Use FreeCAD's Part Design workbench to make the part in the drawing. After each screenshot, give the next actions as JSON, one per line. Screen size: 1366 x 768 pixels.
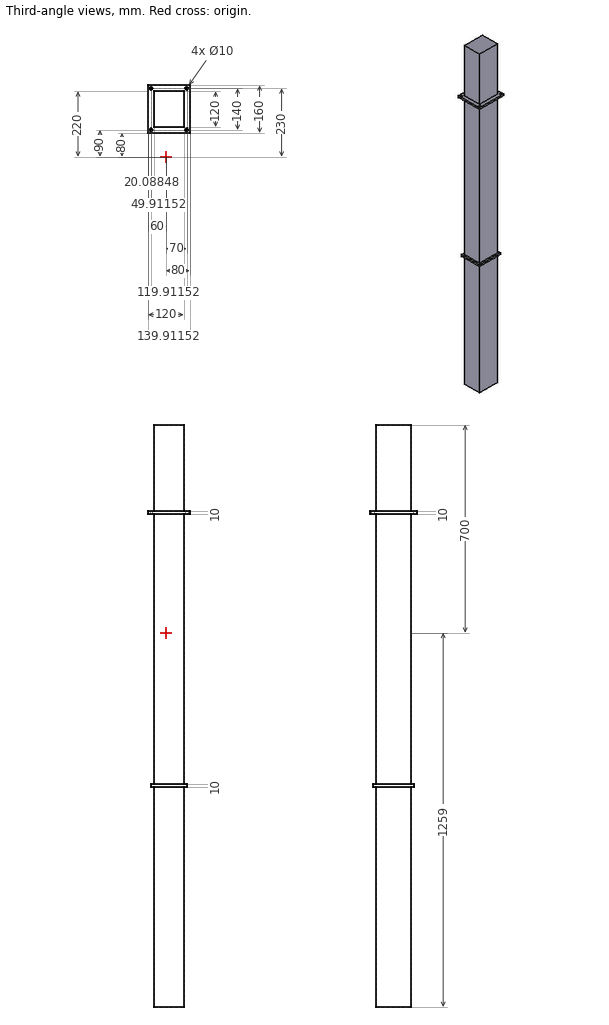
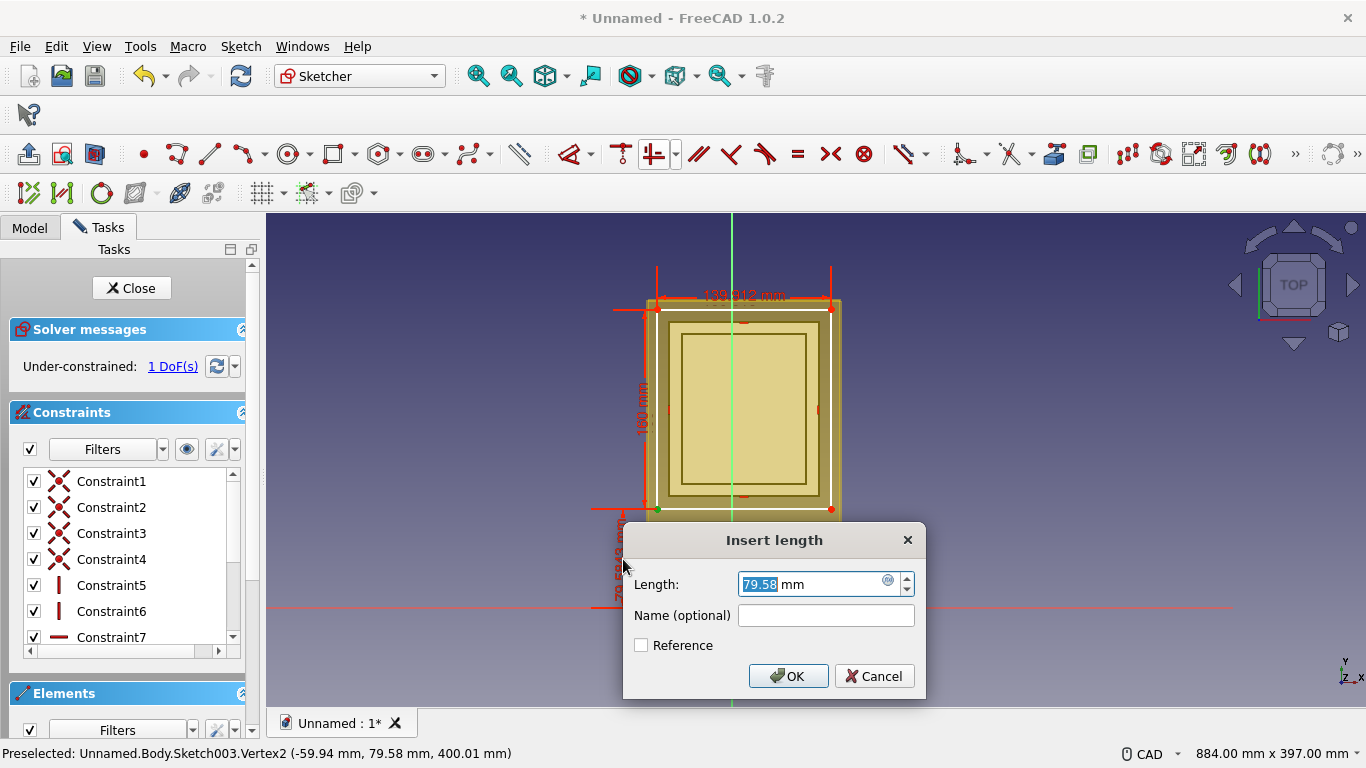
{"action": "type", "text": "80"}
{"action": "key", "text": "Return"}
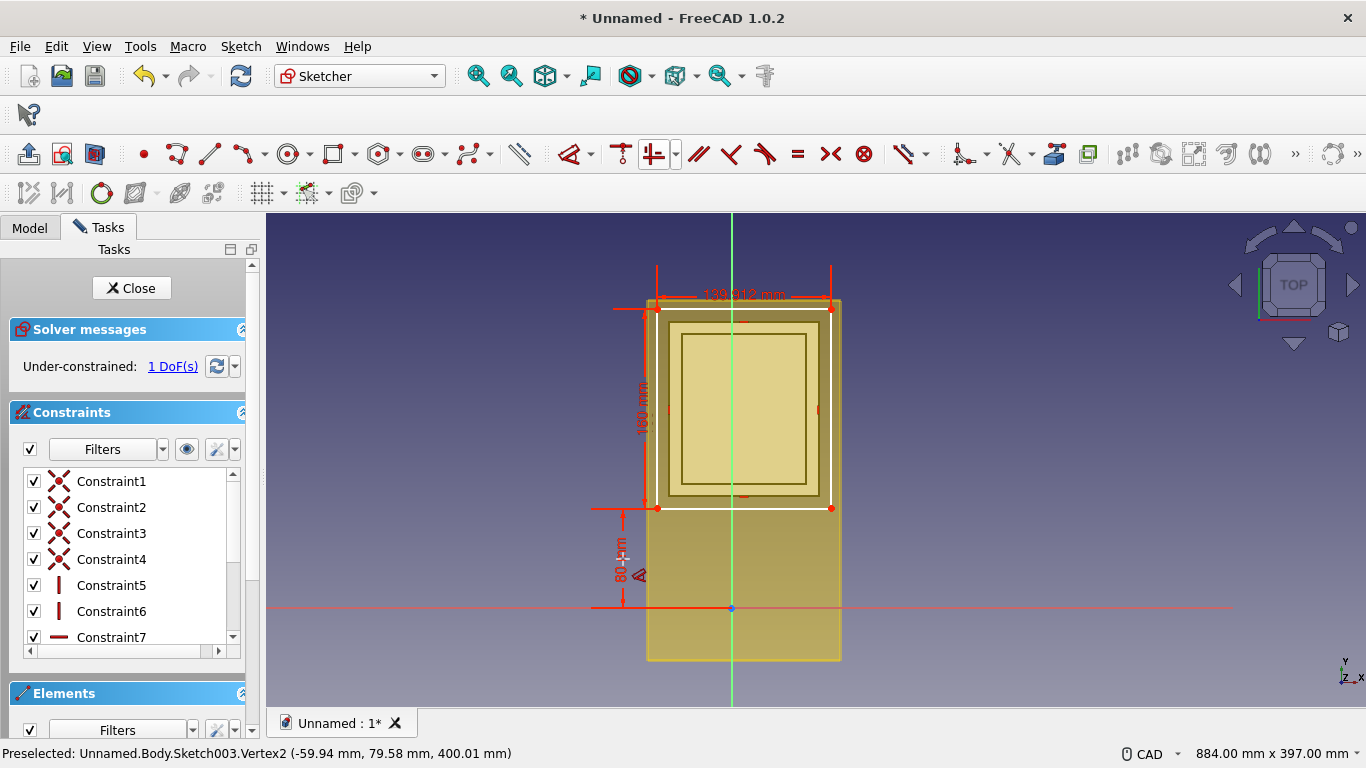
{"action": "left_click", "coordinate": [831, 509]}
{"action": "left_click", "coordinate": [781, 642]}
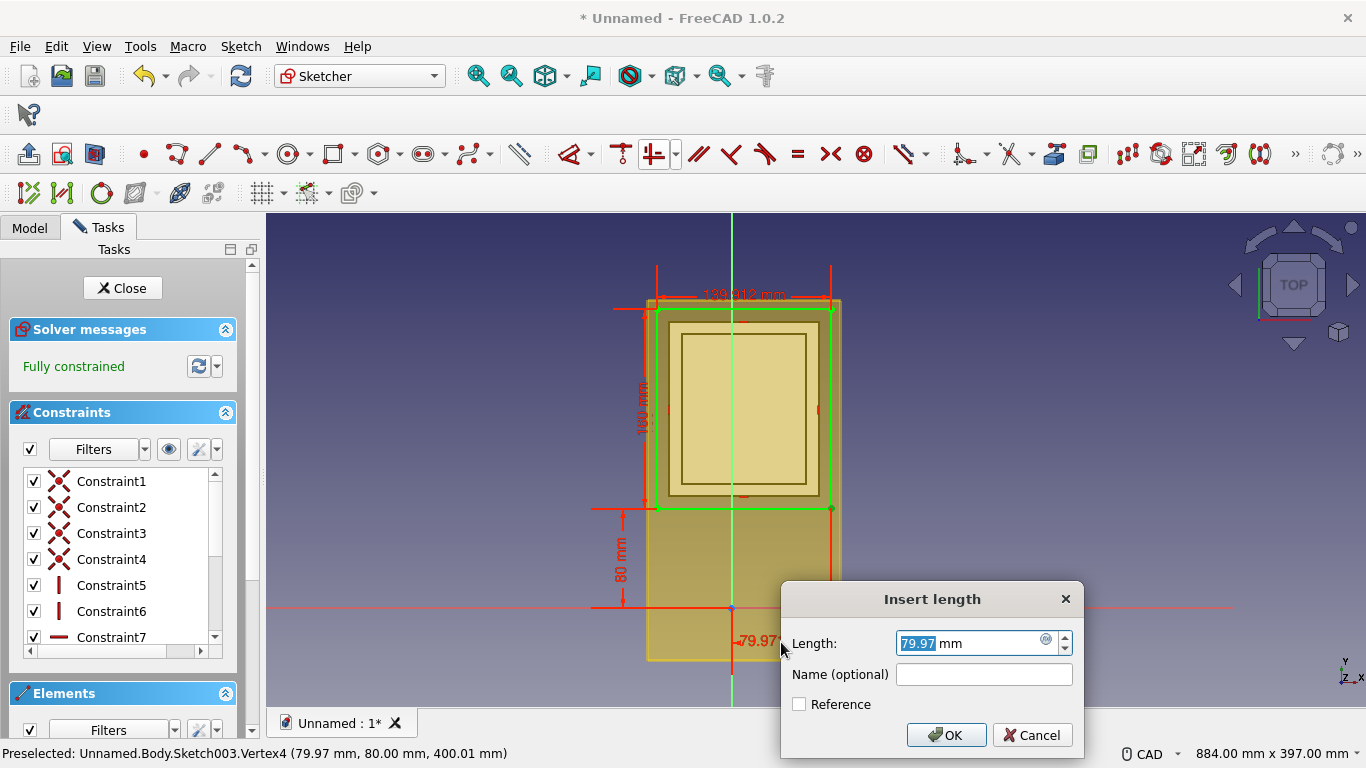
{"action": "type", "text": "80"}
{"action": "key", "text": "Return"}
{"action": "key", "text": "Escape"}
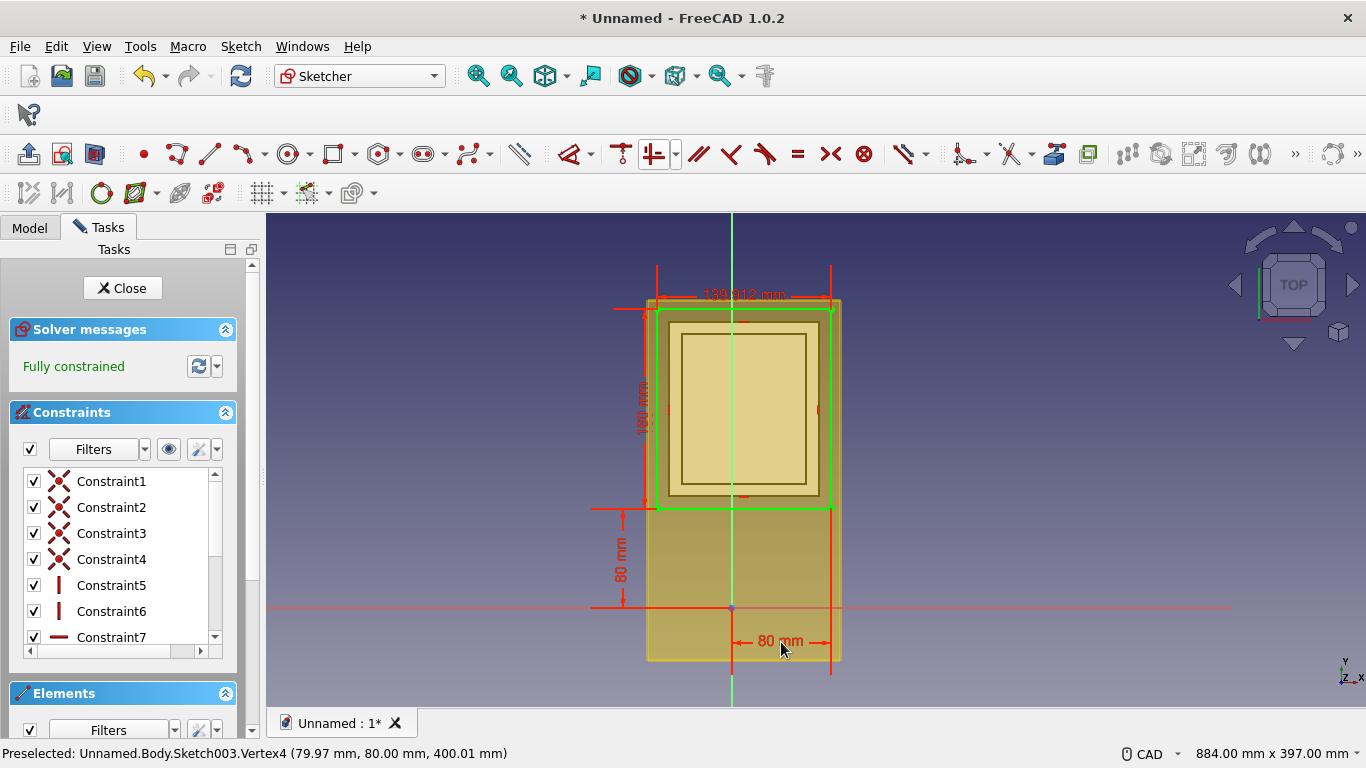
{"action": "left_click", "coordinate": [123, 288]}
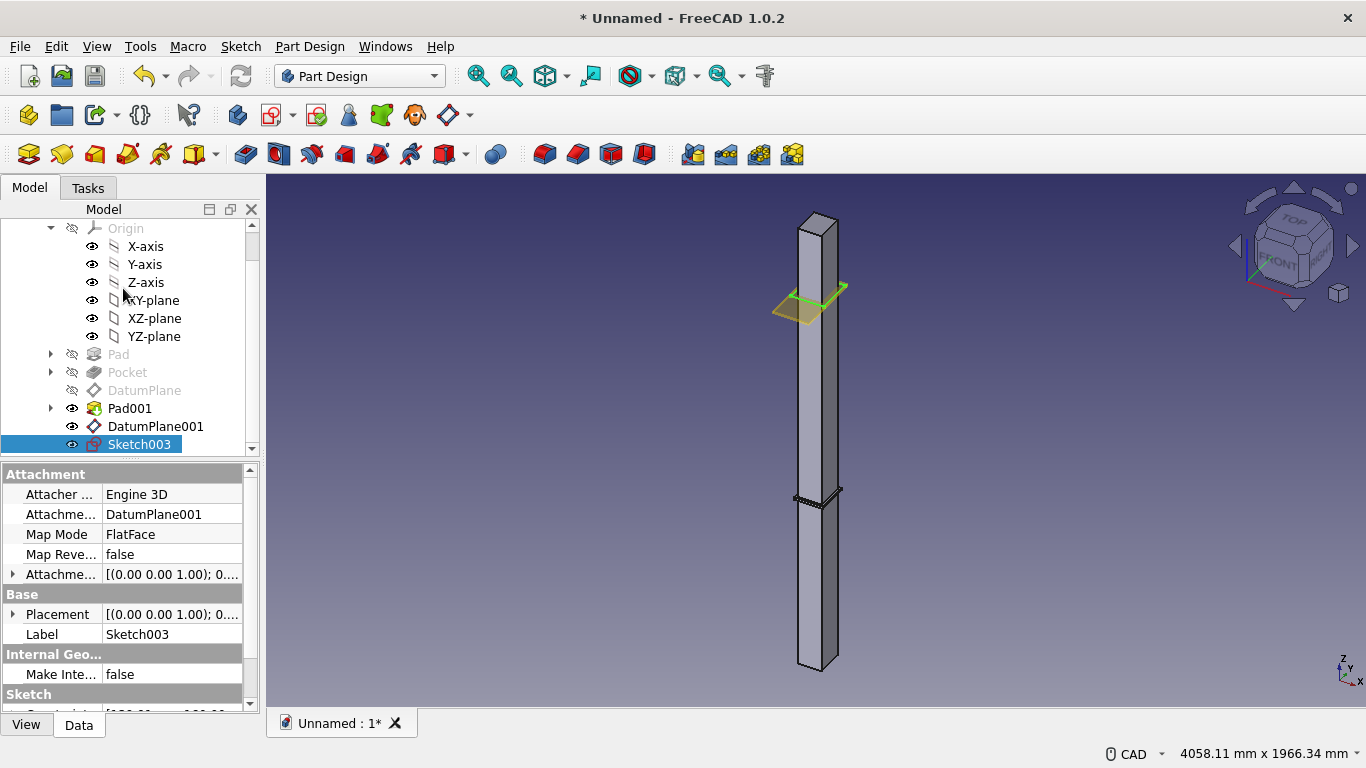
{"action": "left_click", "coordinate": [29, 154]}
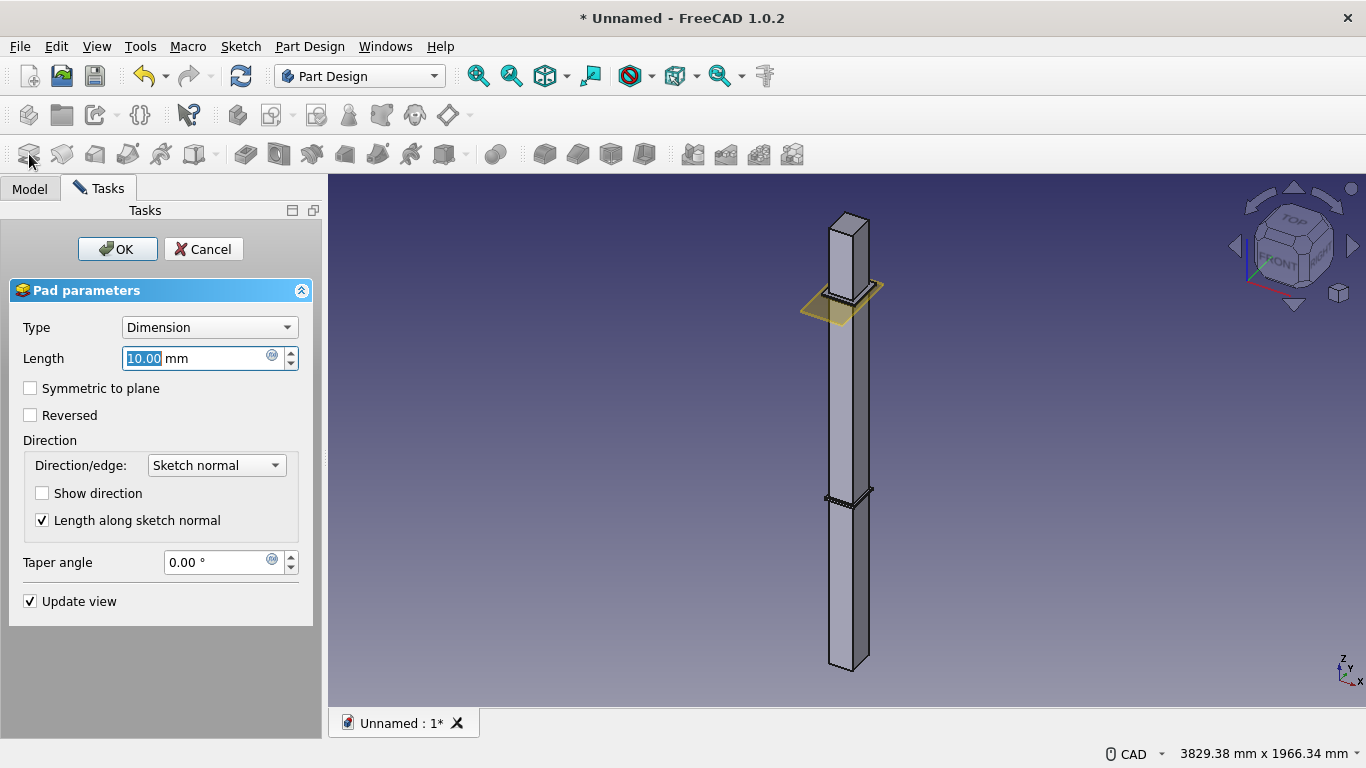
{"action": "type", "text": "10"}
{"action": "key", "text": "Tab"}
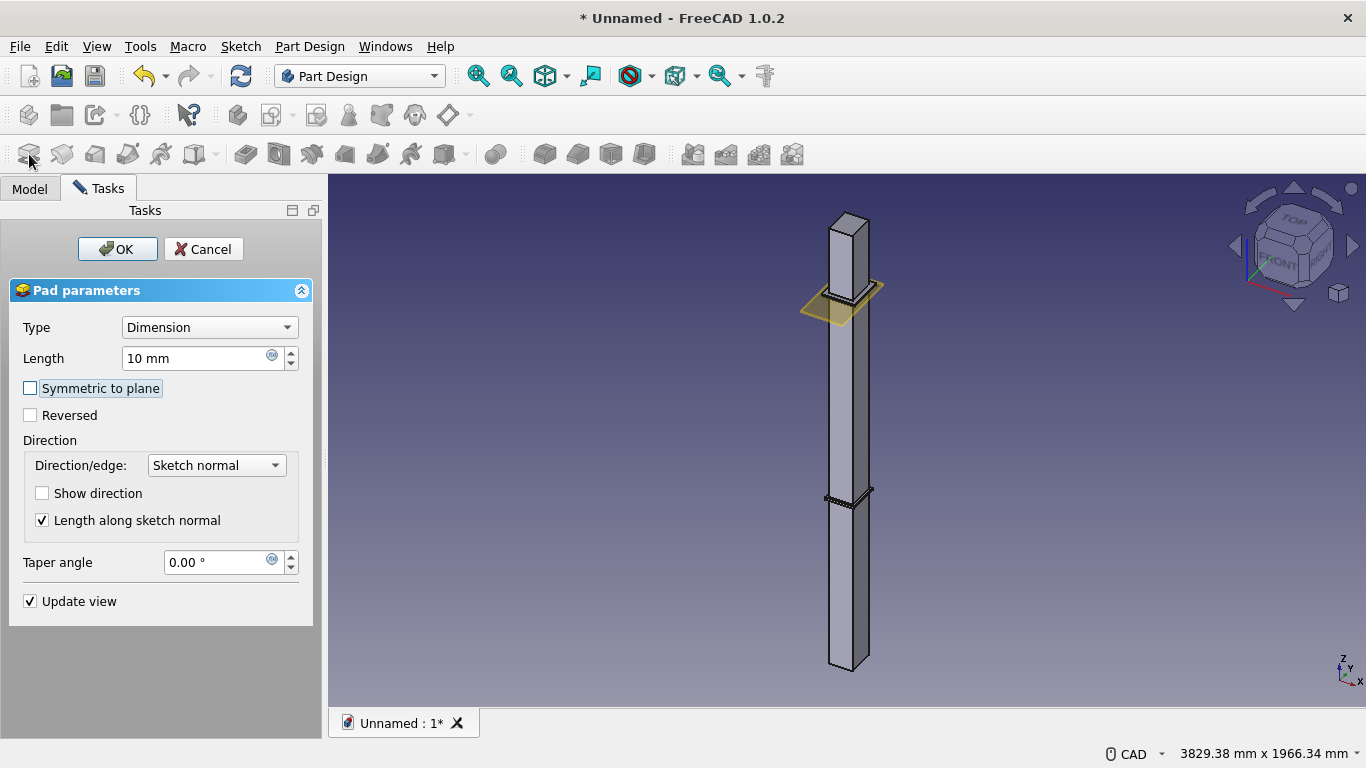
{"action": "left_click", "coordinate": [118, 249]}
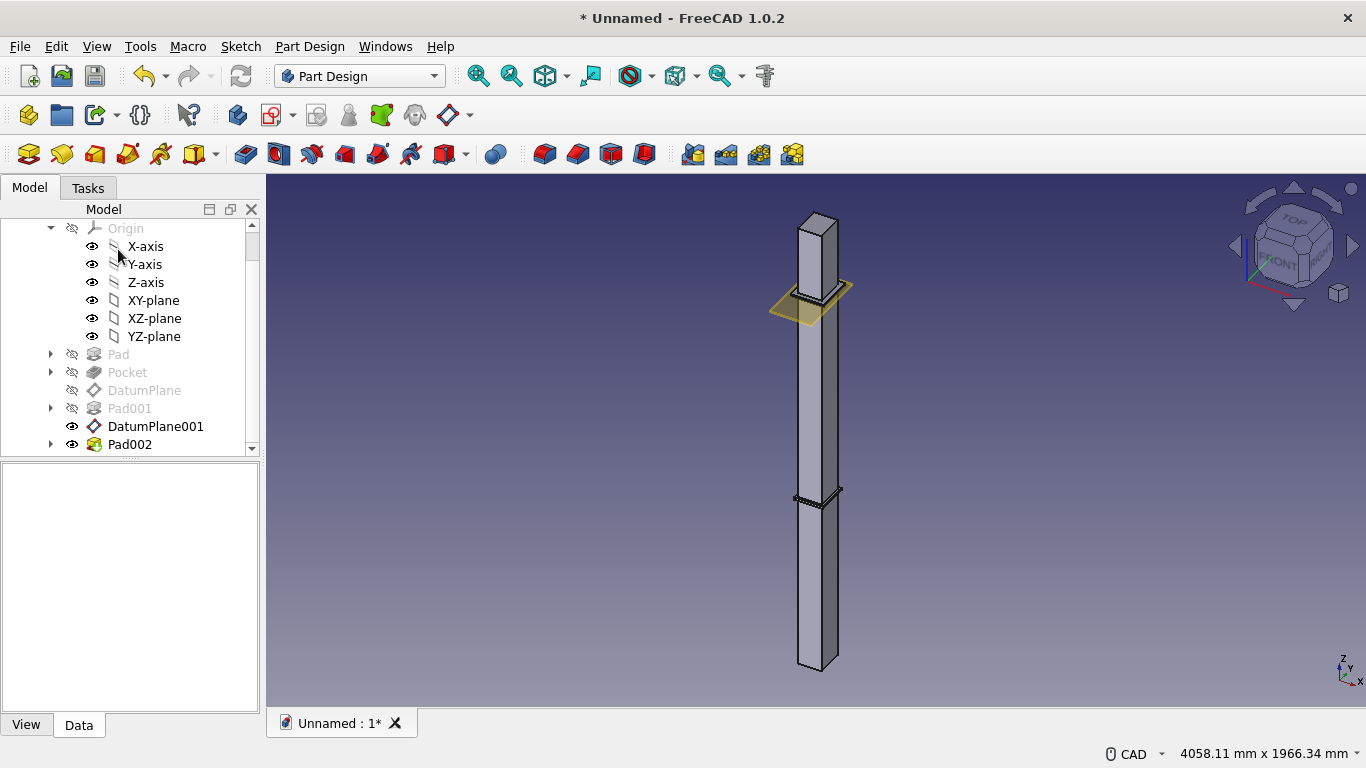
{"action": "left_click", "coordinate": [117, 426]}
{"action": "key", "text": "space"}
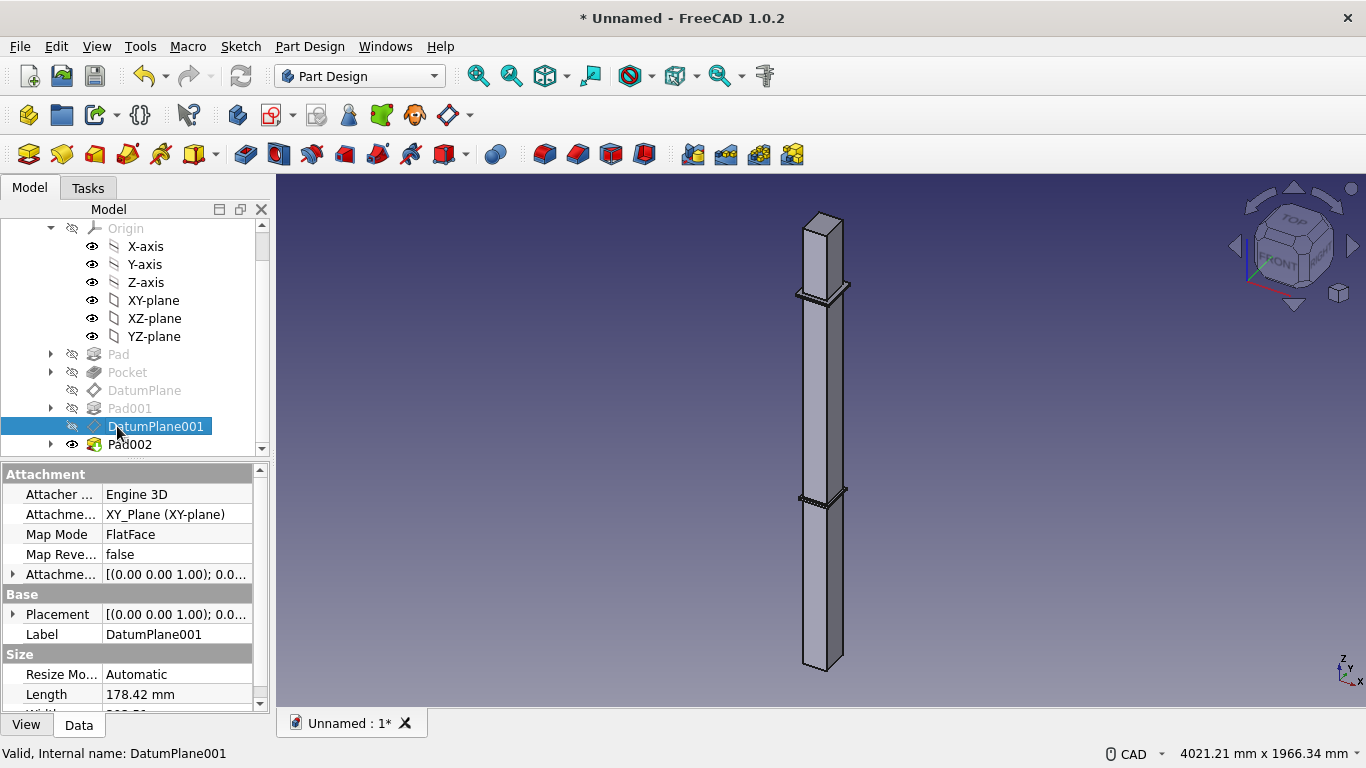
{"action": "scroll", "coordinate": [818, 274], "scroll_direction": "up", "scroll_amount": 8}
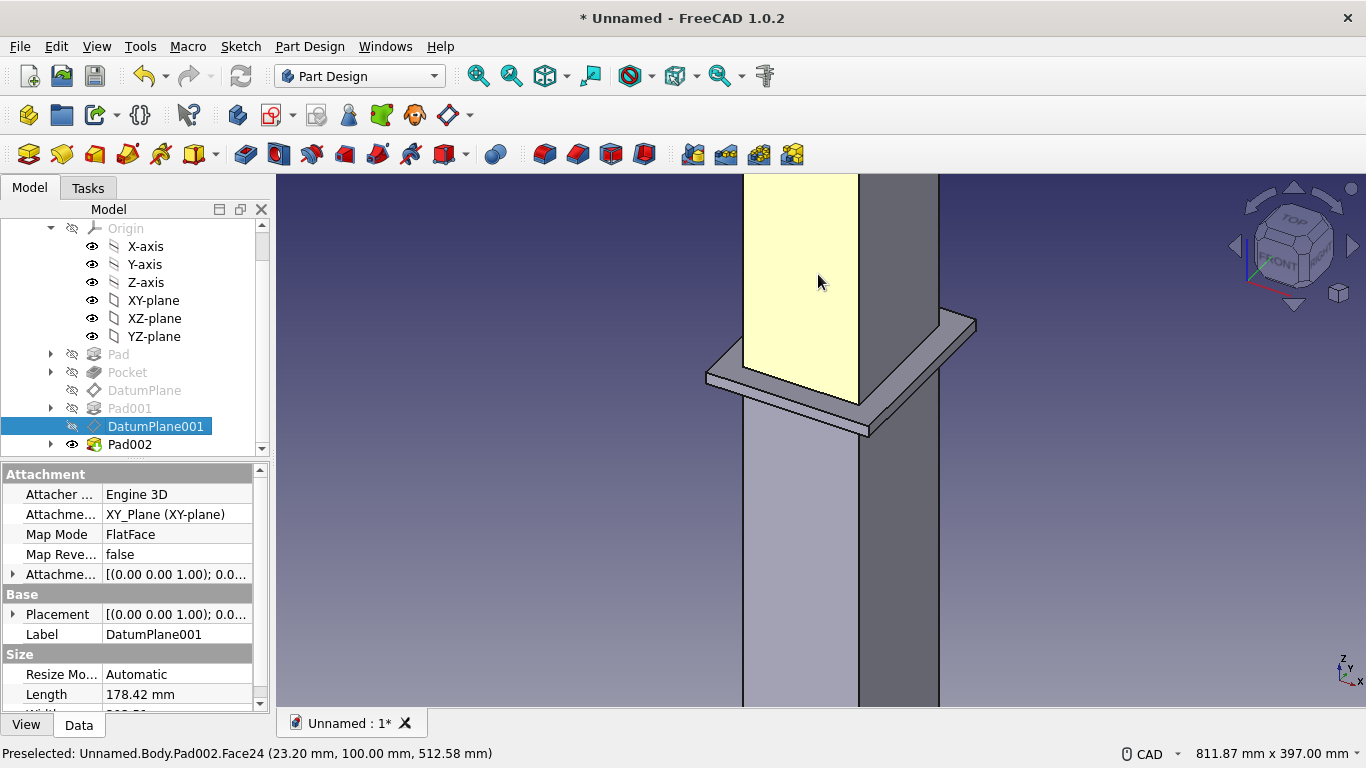
{"action": "left_click", "coordinate": [725, 368]}